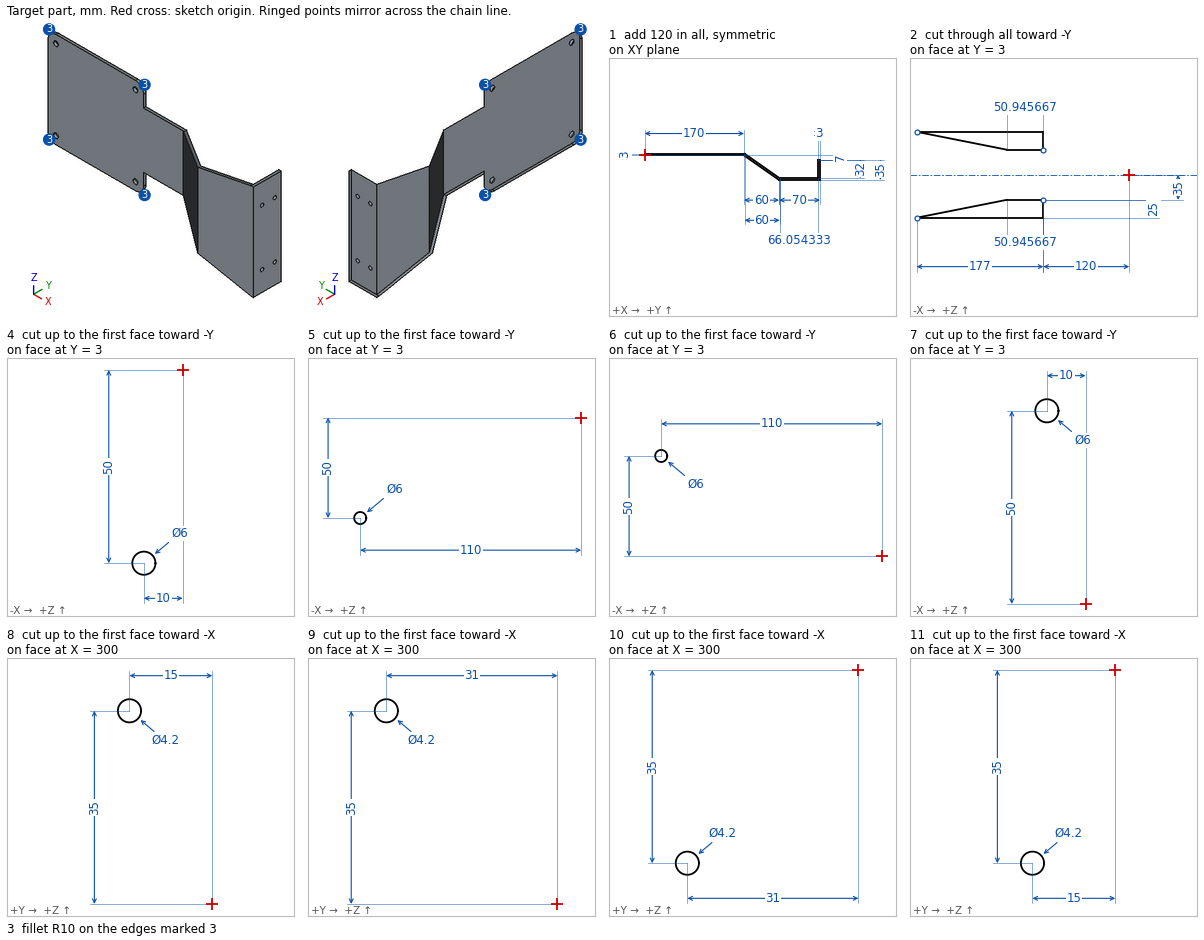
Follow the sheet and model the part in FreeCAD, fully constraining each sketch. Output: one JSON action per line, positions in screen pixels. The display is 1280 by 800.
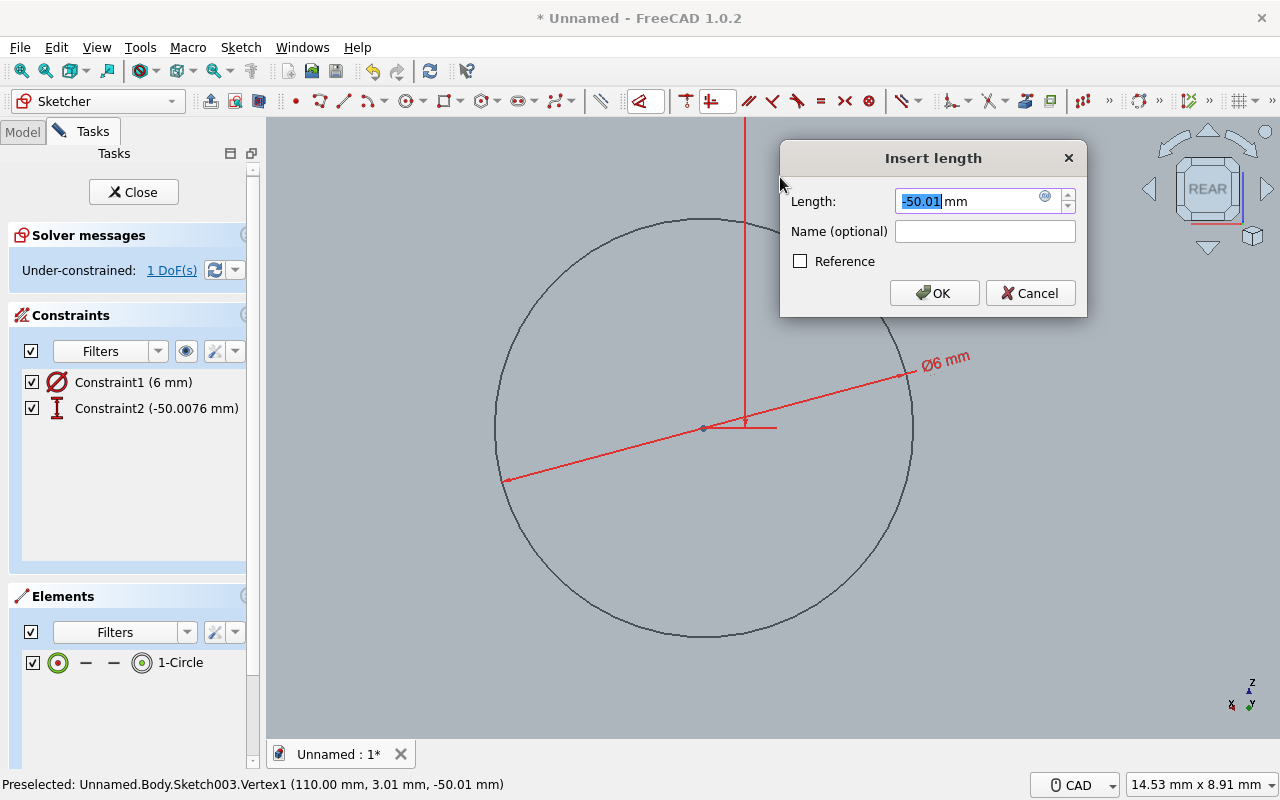
{"action": "type", "text": "-50"}
{"action": "key", "text": "Return"}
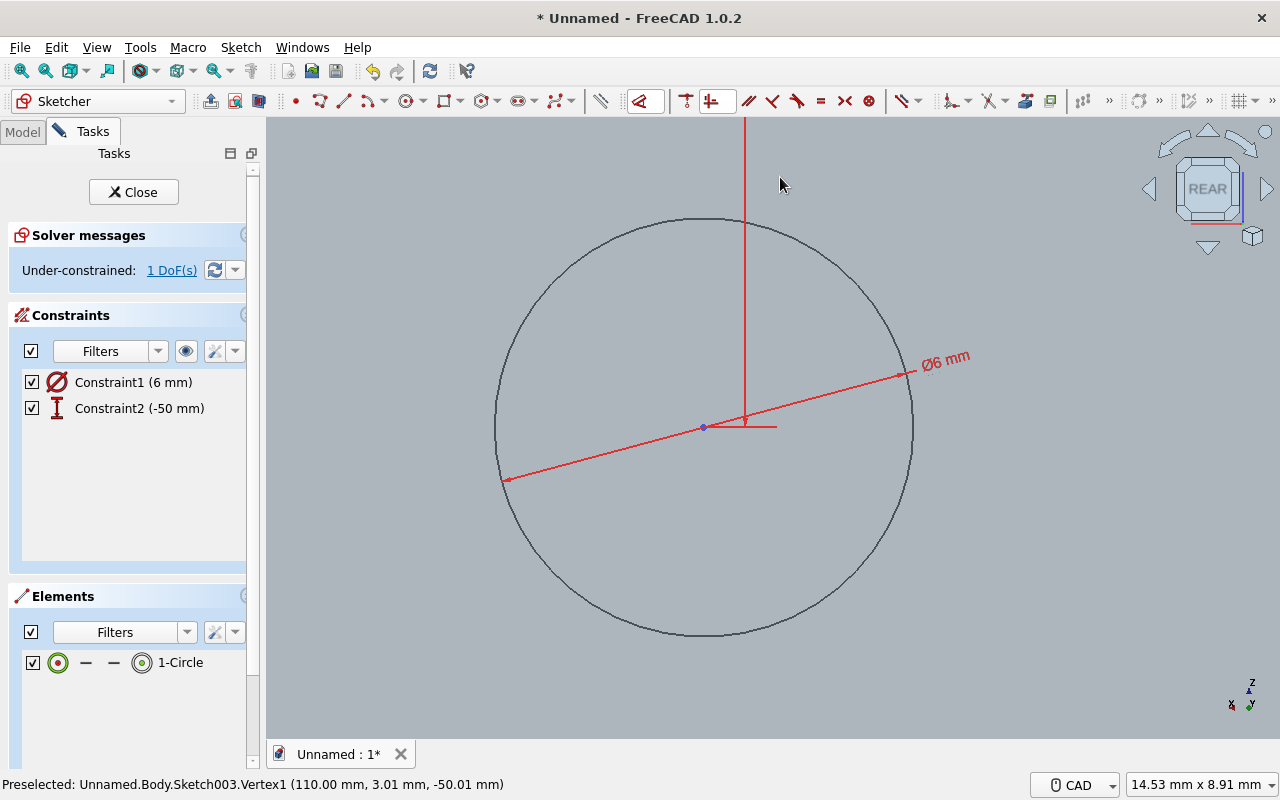
{"action": "left_click", "coordinate": [704, 427]}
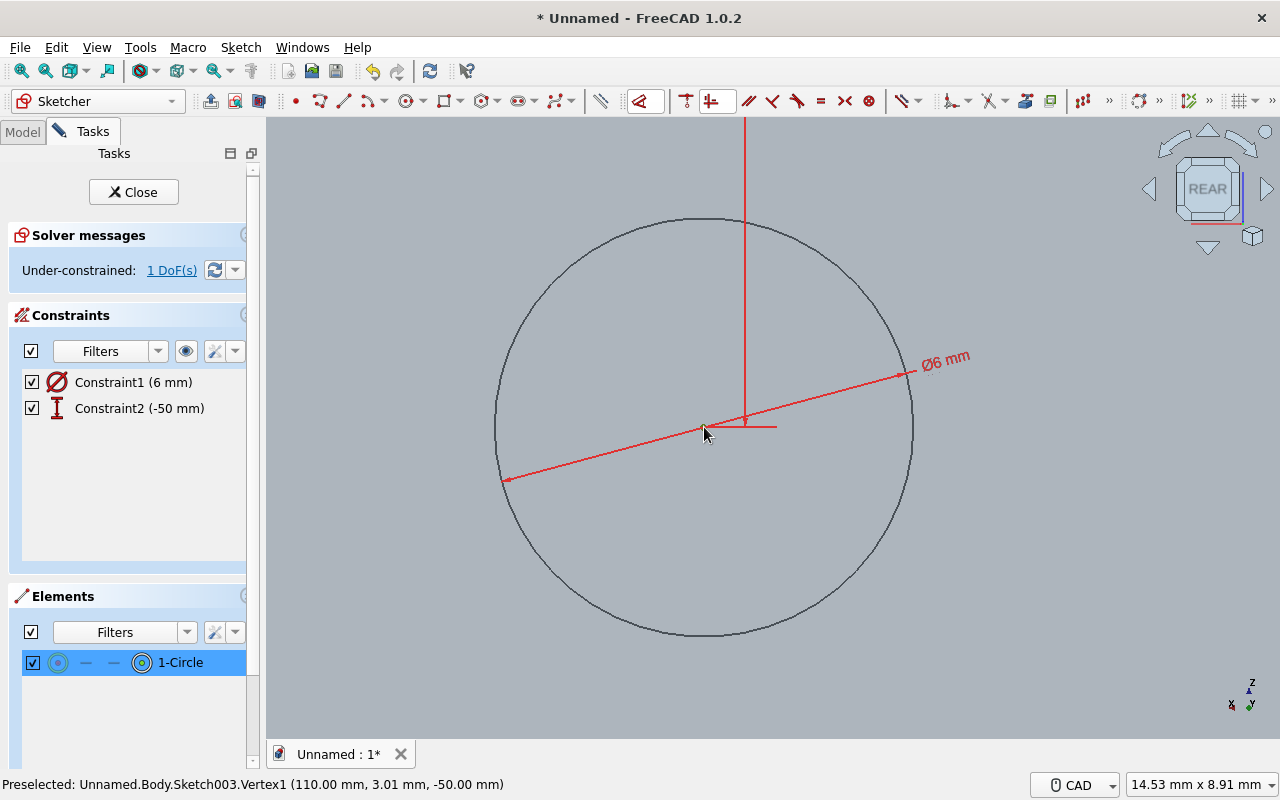
{"action": "left_click", "coordinate": [658, 102]}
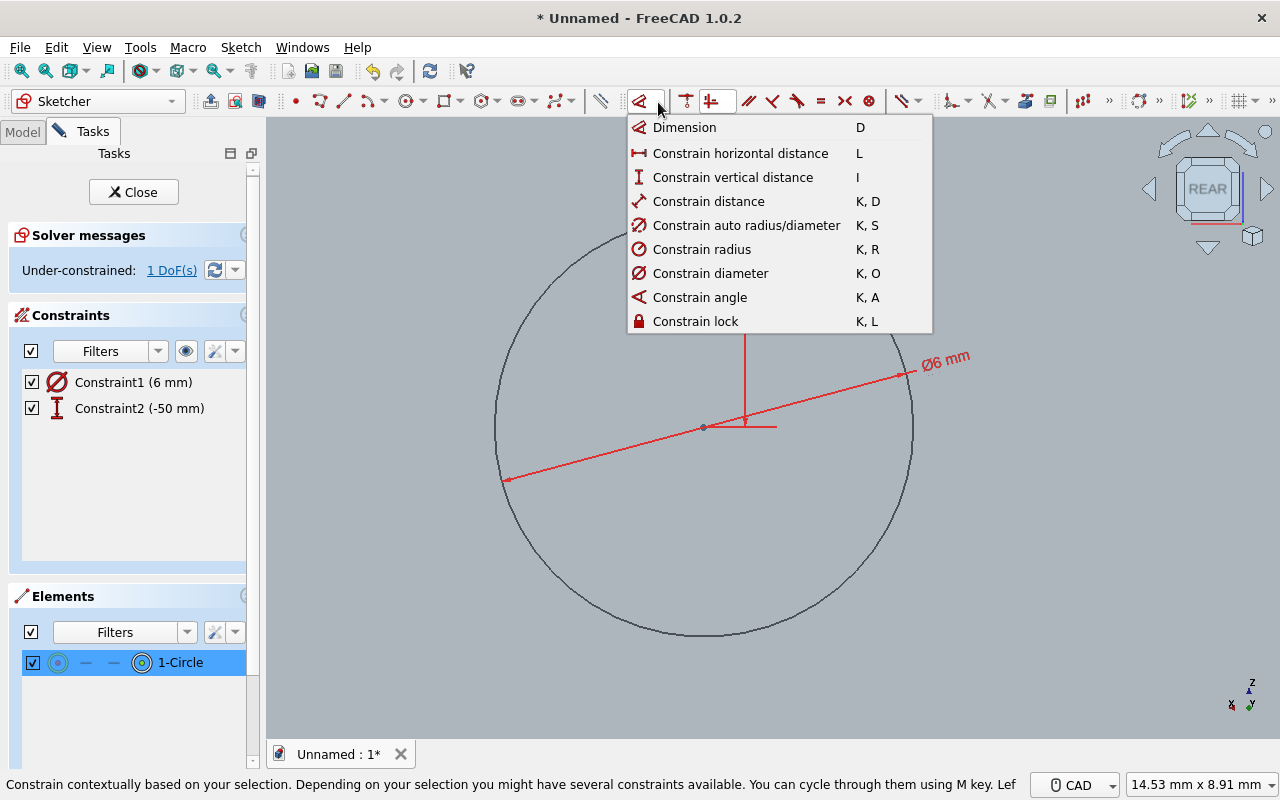
{"action": "left_click", "coordinate": [780, 153]}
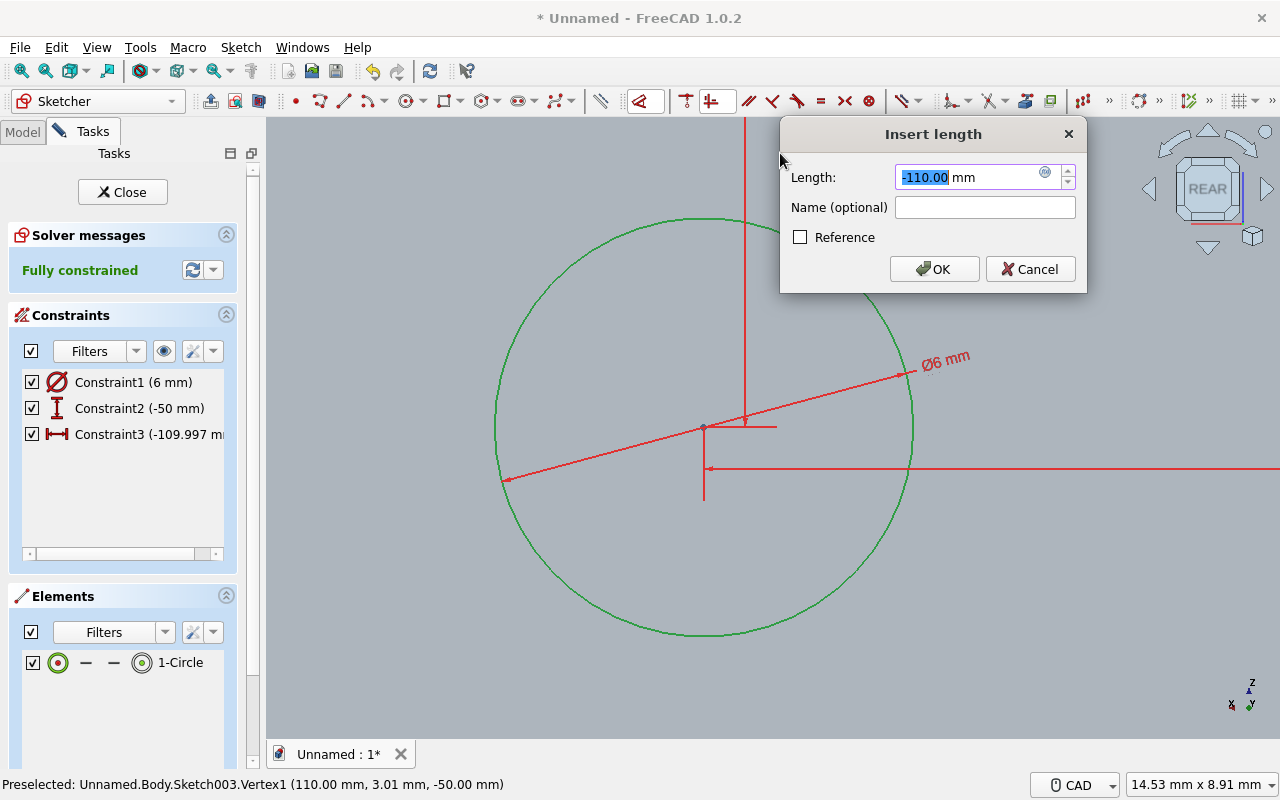
{"action": "type", "text": "-110"}
{"action": "key", "text": "Return"}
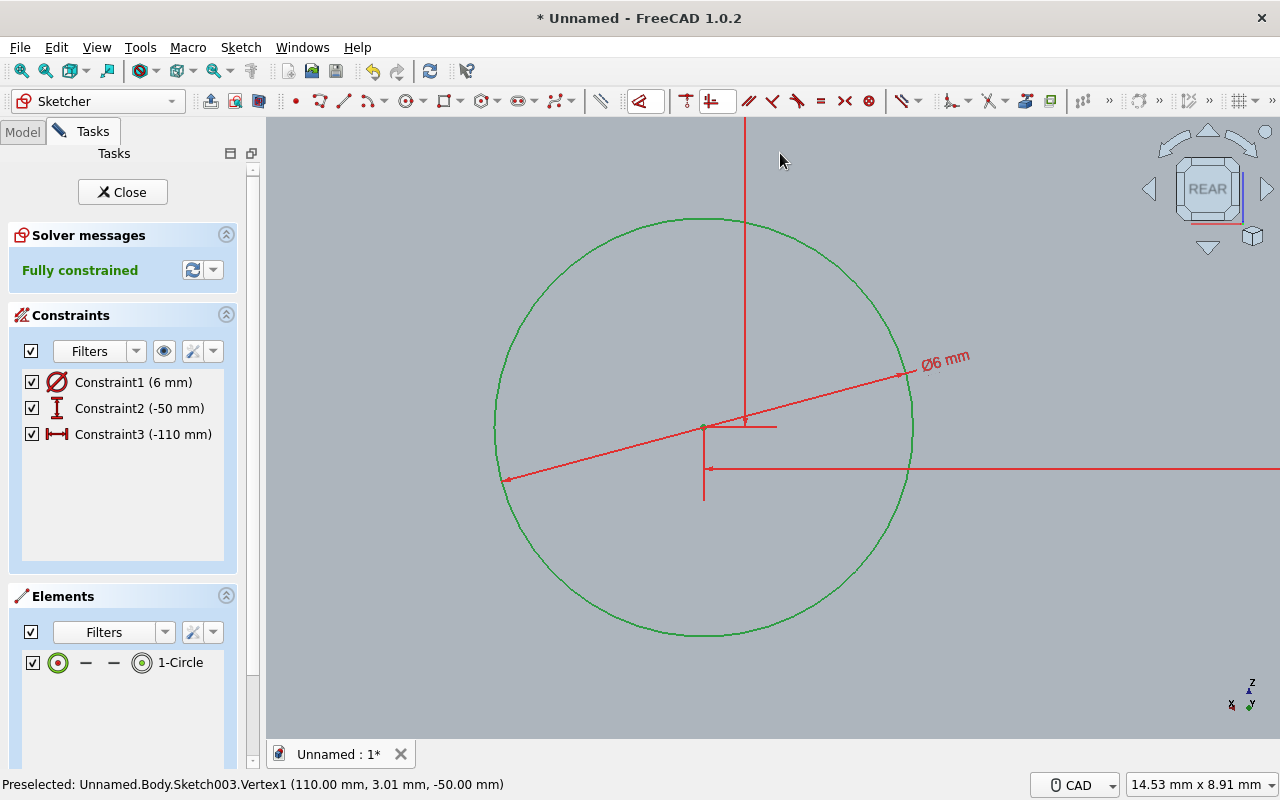
{"action": "left_click", "coordinate": [123, 192]}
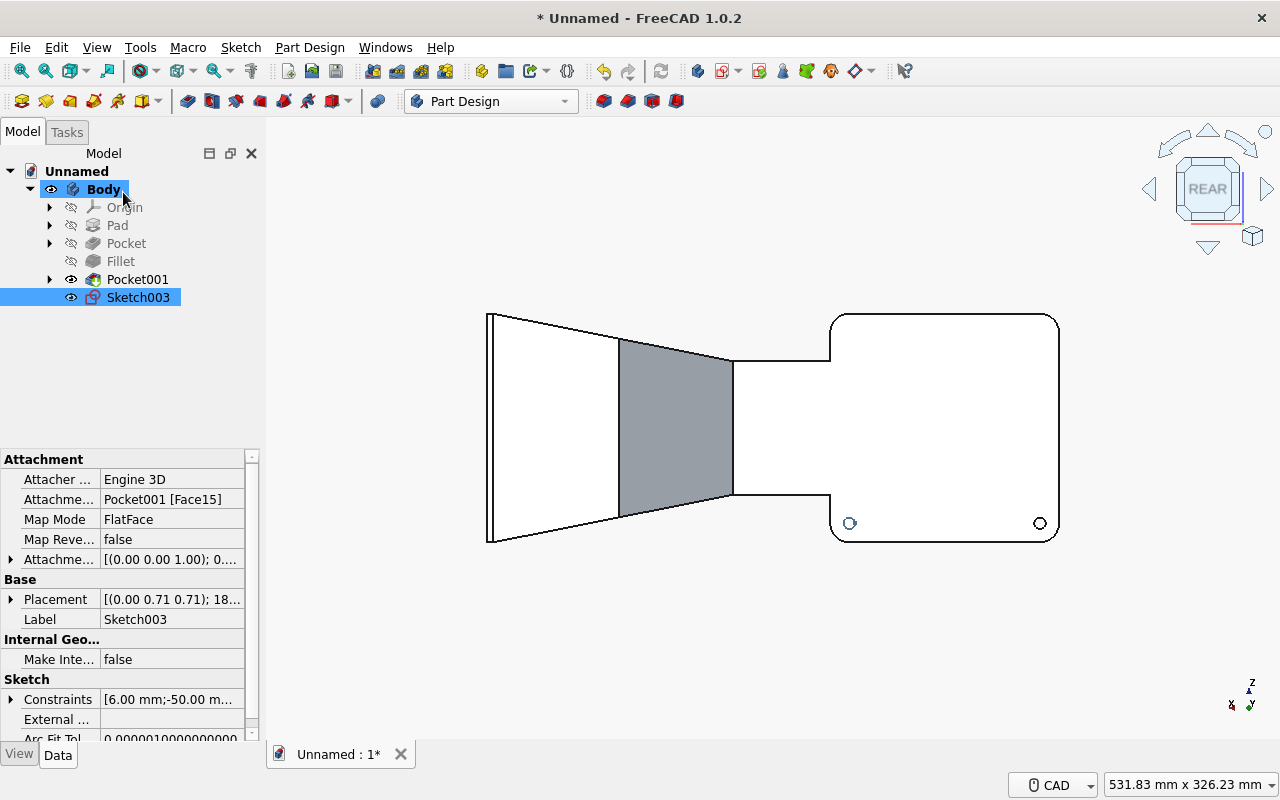
{"action": "left_click", "coordinate": [188, 102]}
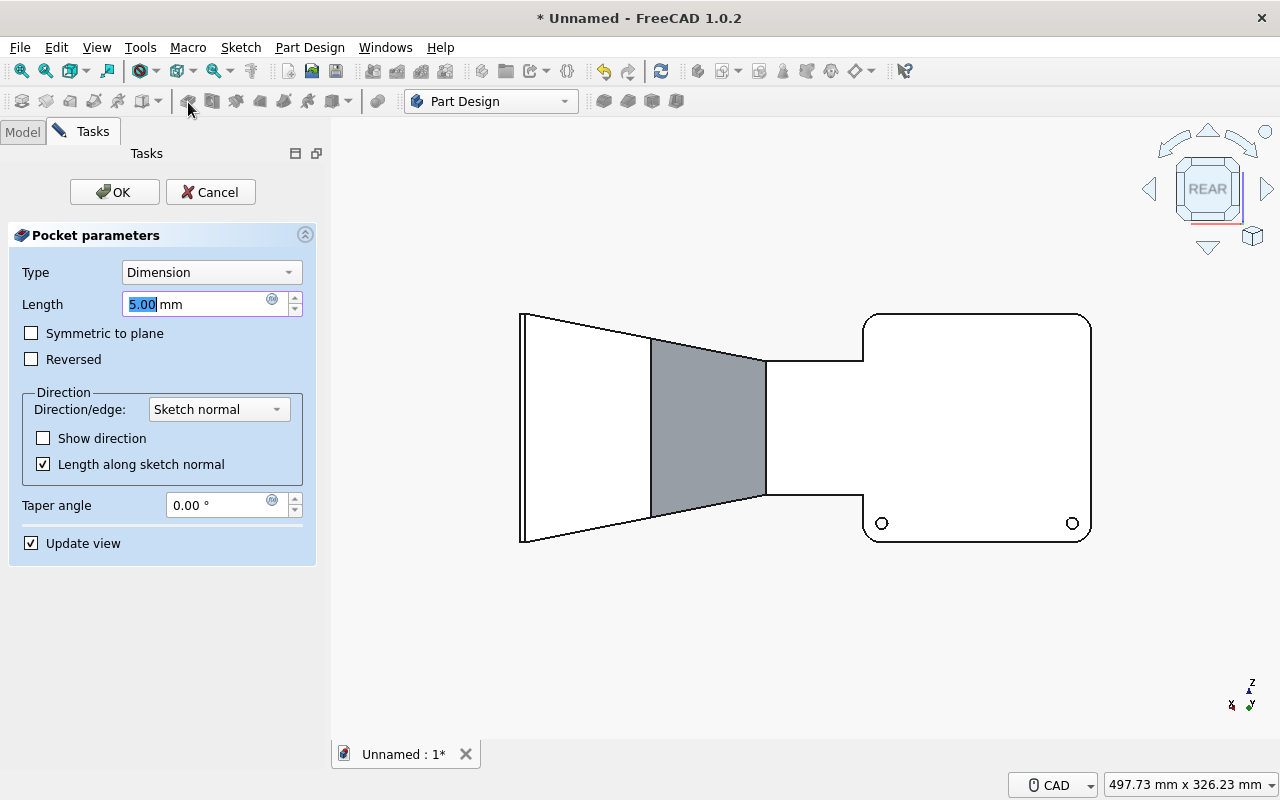
{"action": "left_click", "coordinate": [212, 272]}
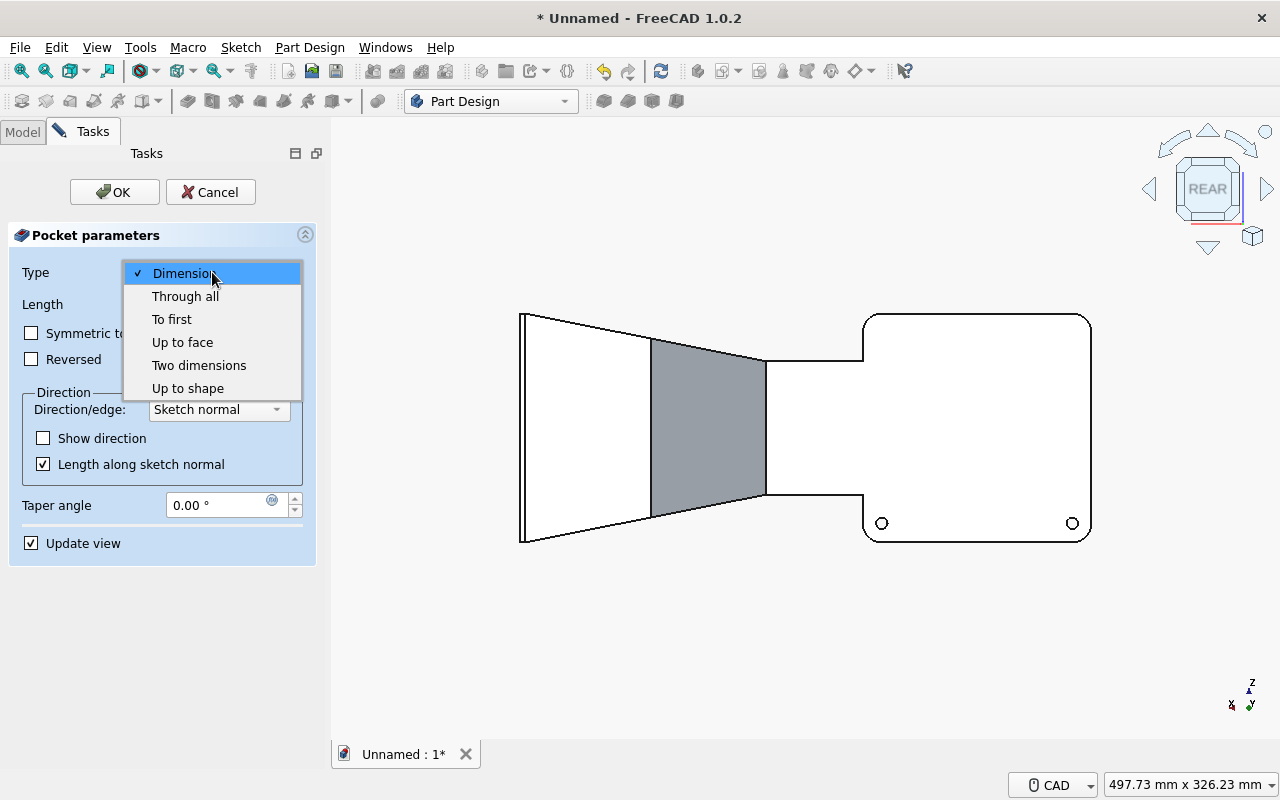
{"action": "left_click", "coordinate": [212, 320]}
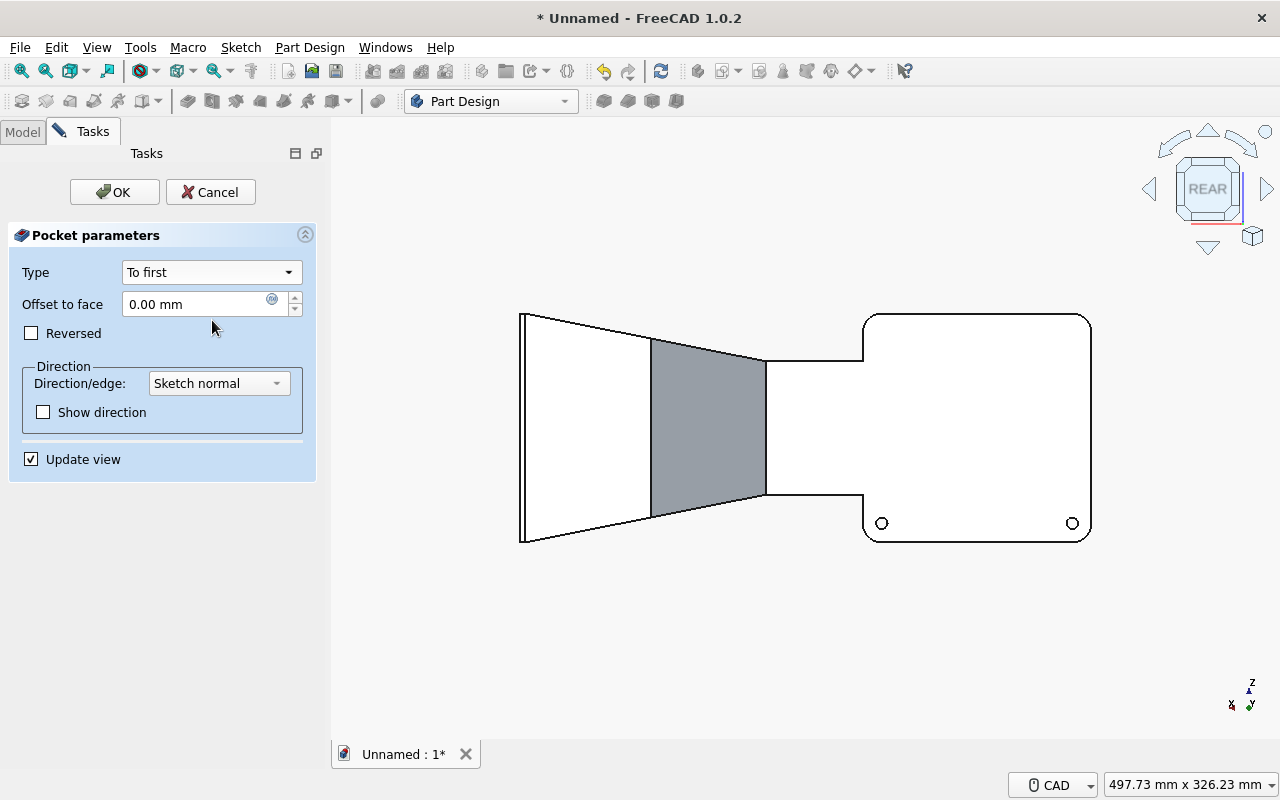
{"action": "left_click", "coordinate": [115, 192]}